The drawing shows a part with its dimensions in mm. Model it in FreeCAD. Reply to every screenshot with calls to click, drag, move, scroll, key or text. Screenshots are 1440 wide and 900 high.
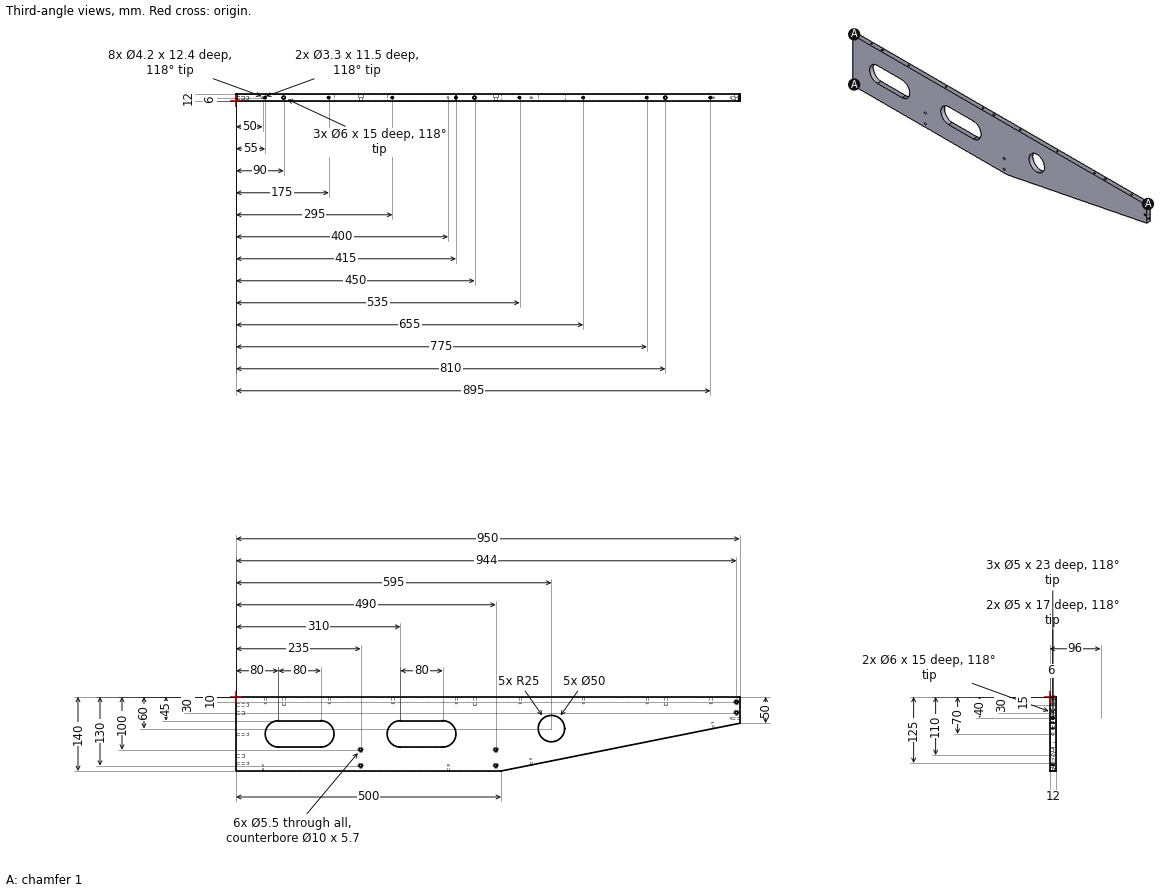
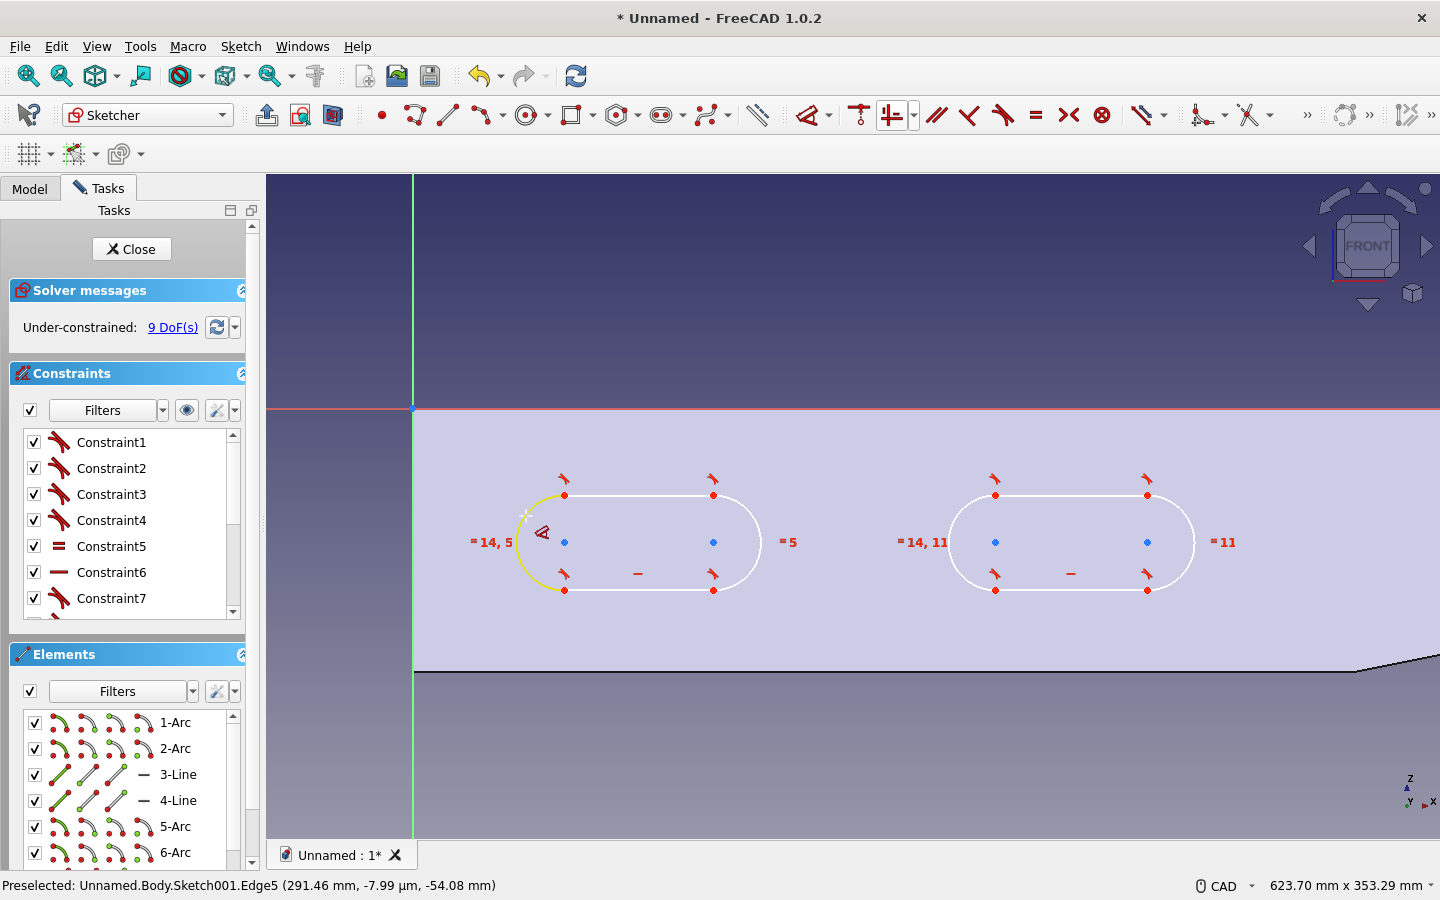
click(526, 515)
click(500, 496)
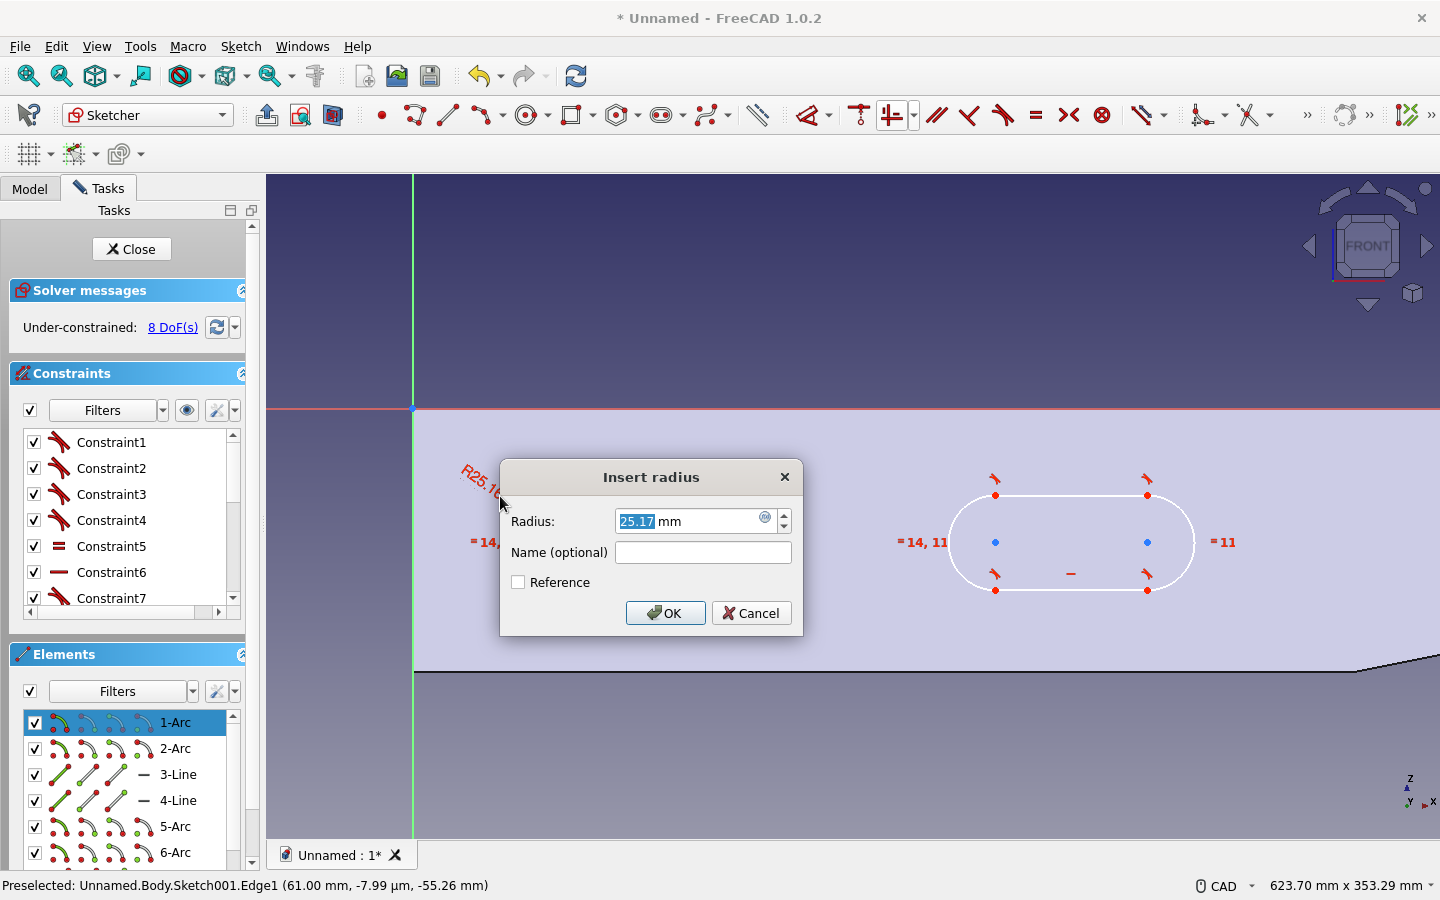
text(25)
key(Return)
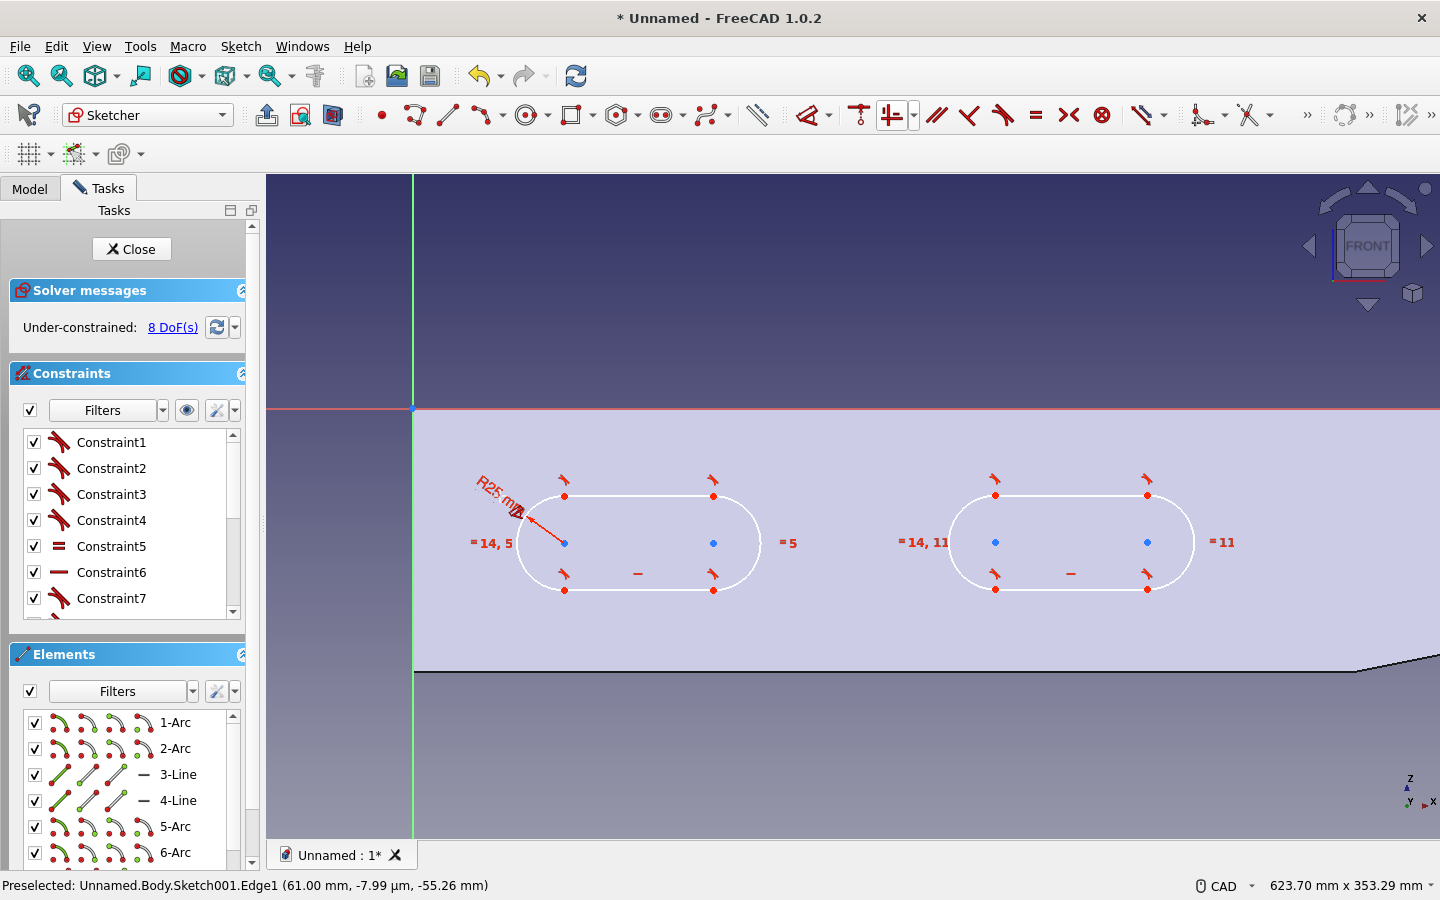
click(609, 496)
click(639, 462)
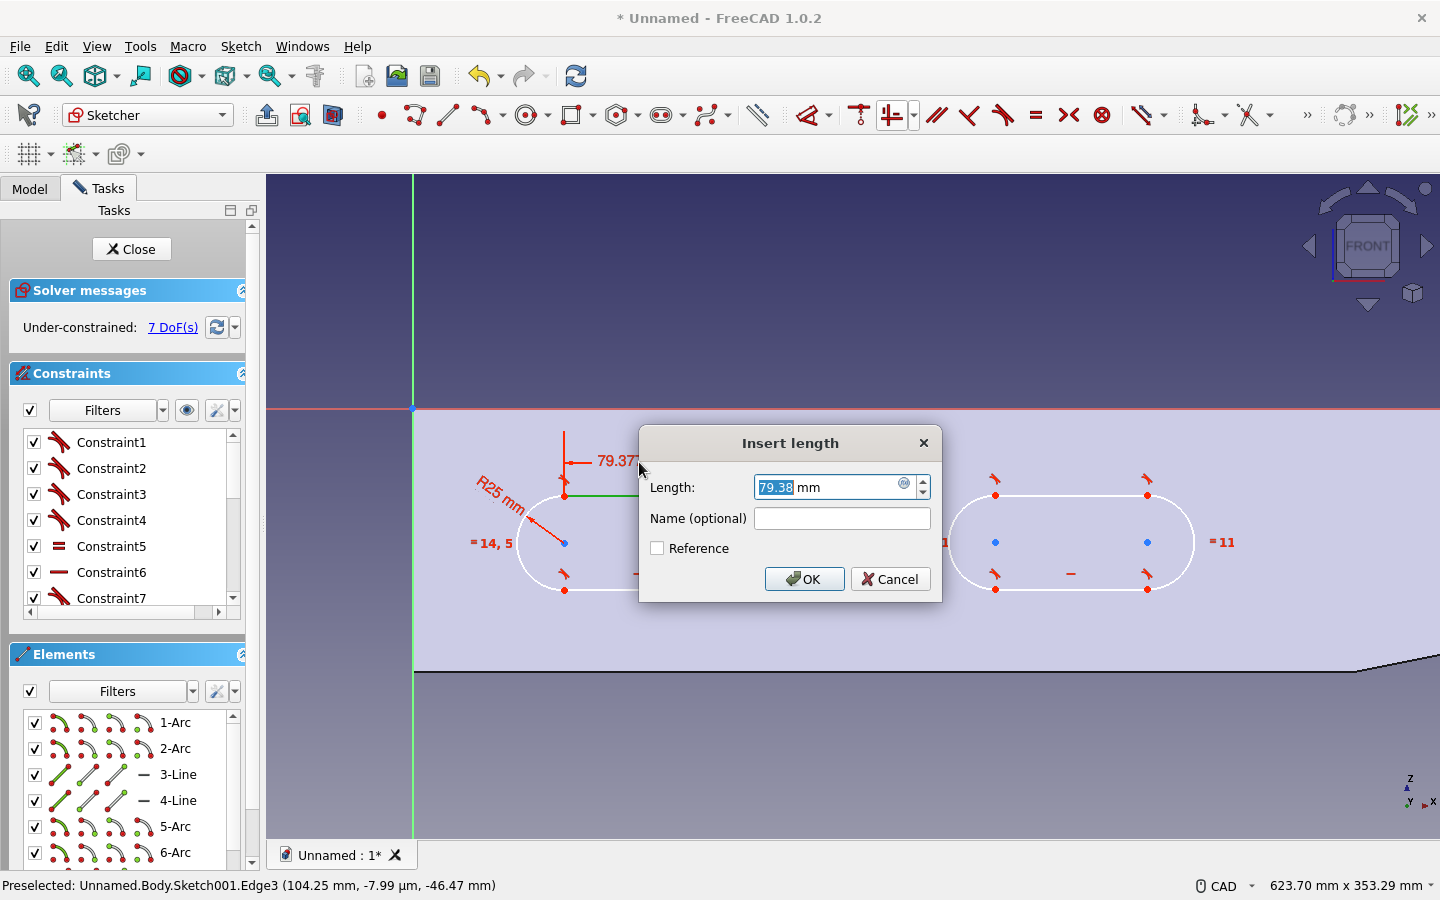
text(80)
key(Return)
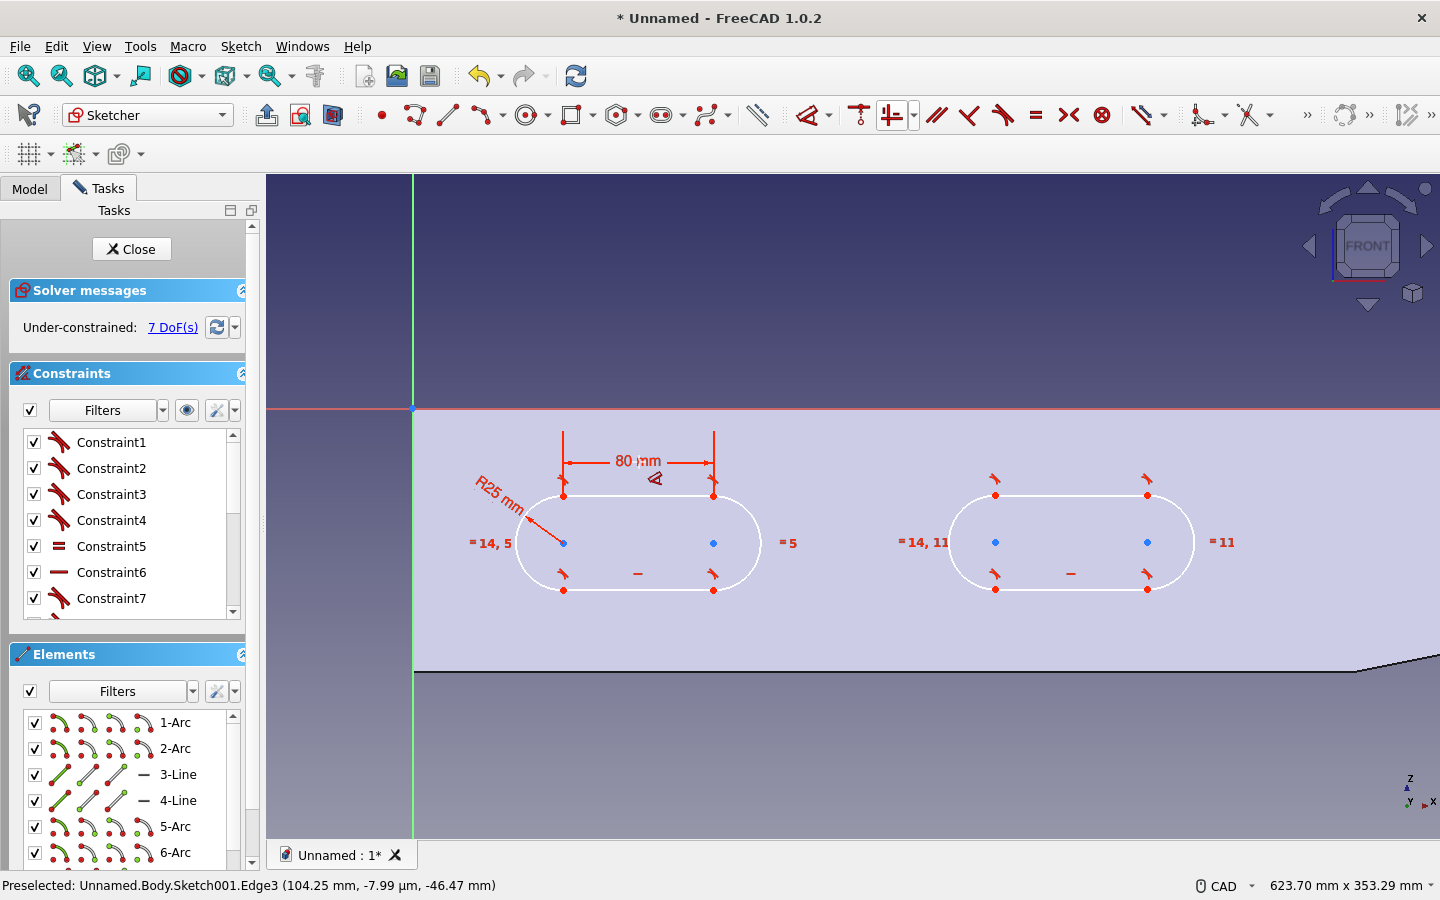
click(1041, 496)
click(1072, 462)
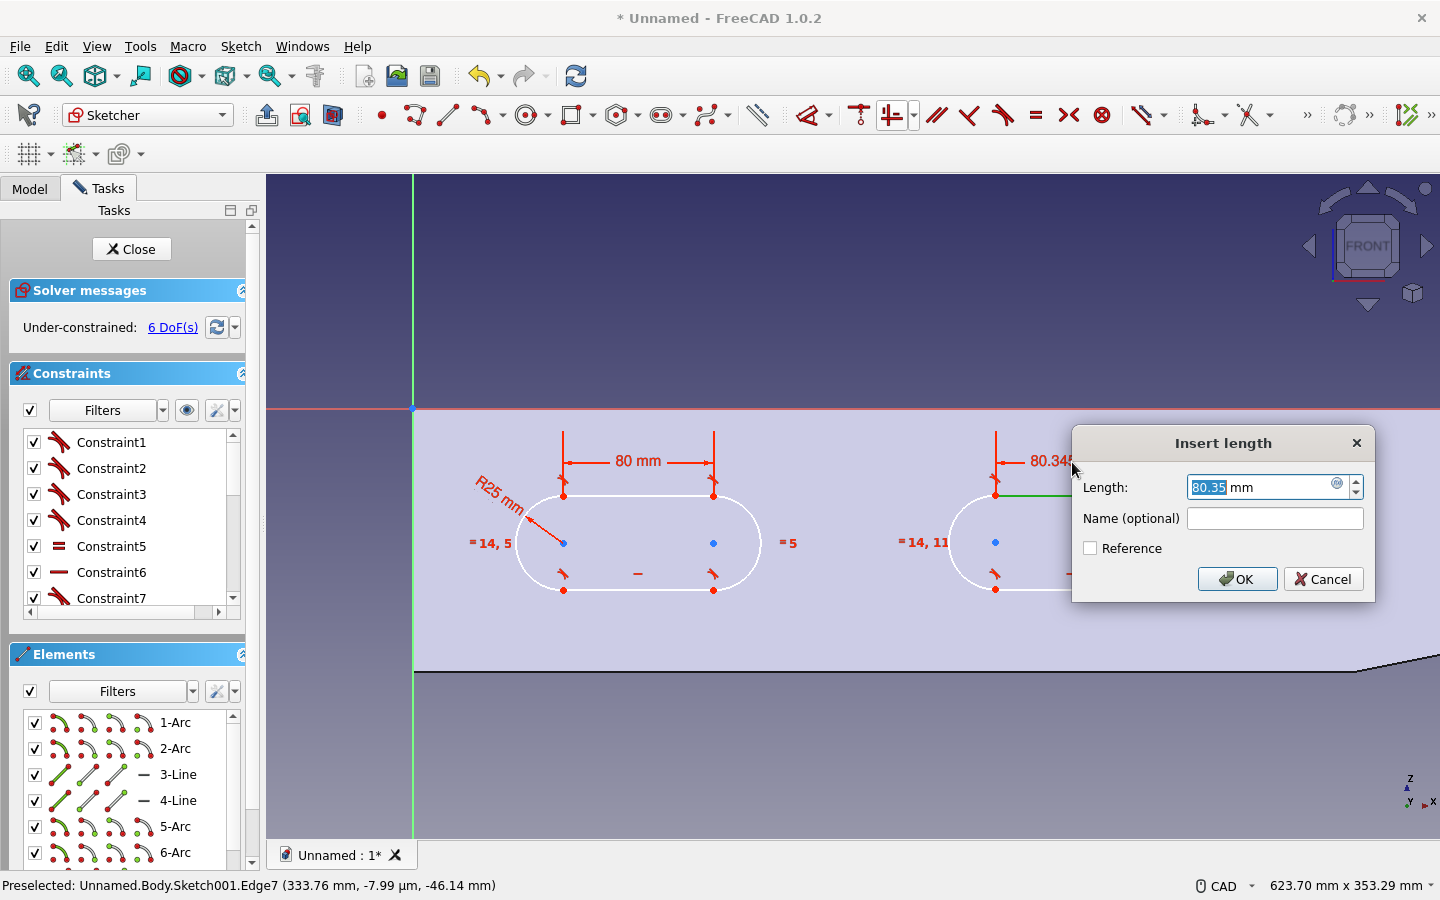
text(80)
key(Return)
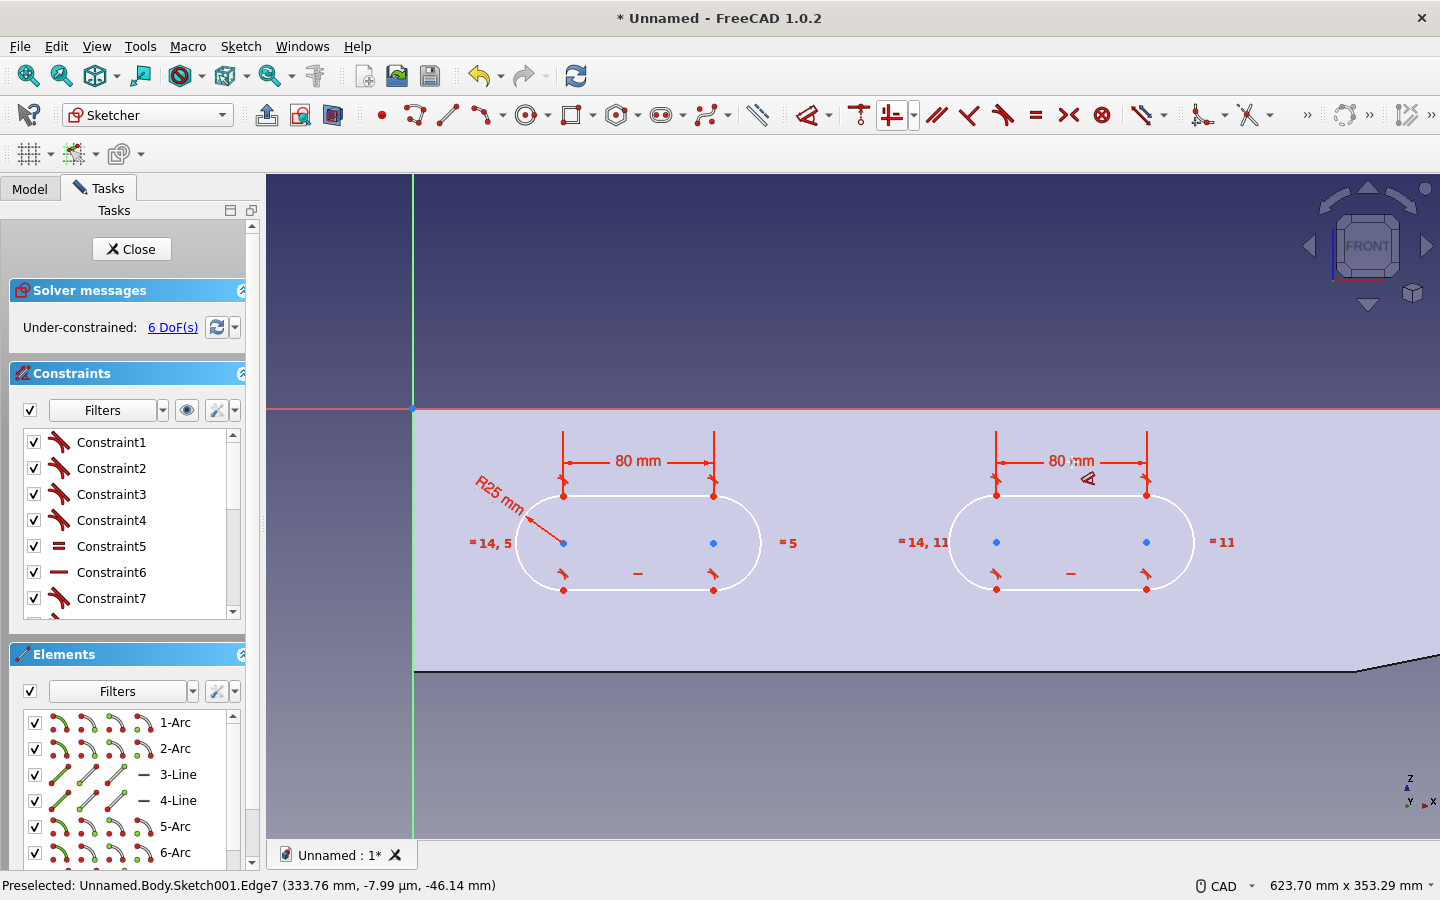
scroll(527, 517, down, 3)